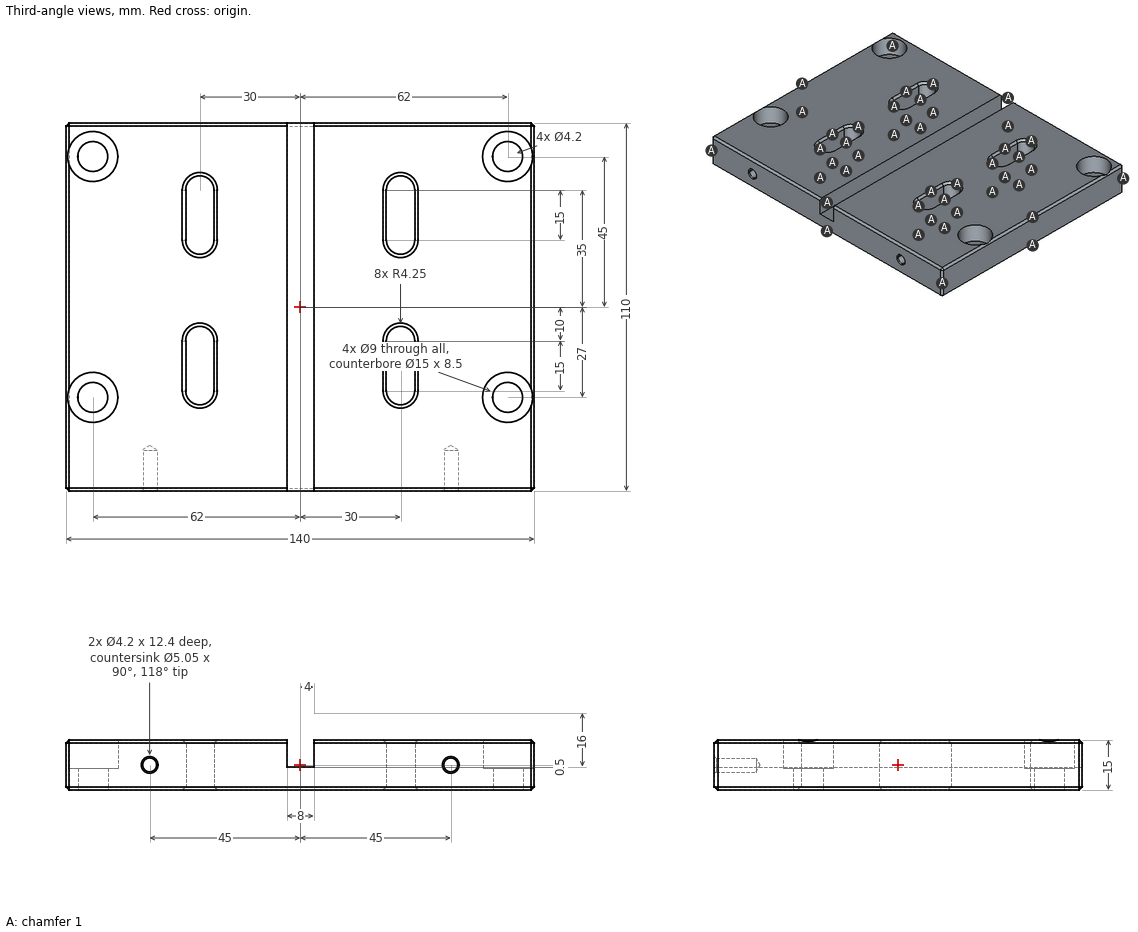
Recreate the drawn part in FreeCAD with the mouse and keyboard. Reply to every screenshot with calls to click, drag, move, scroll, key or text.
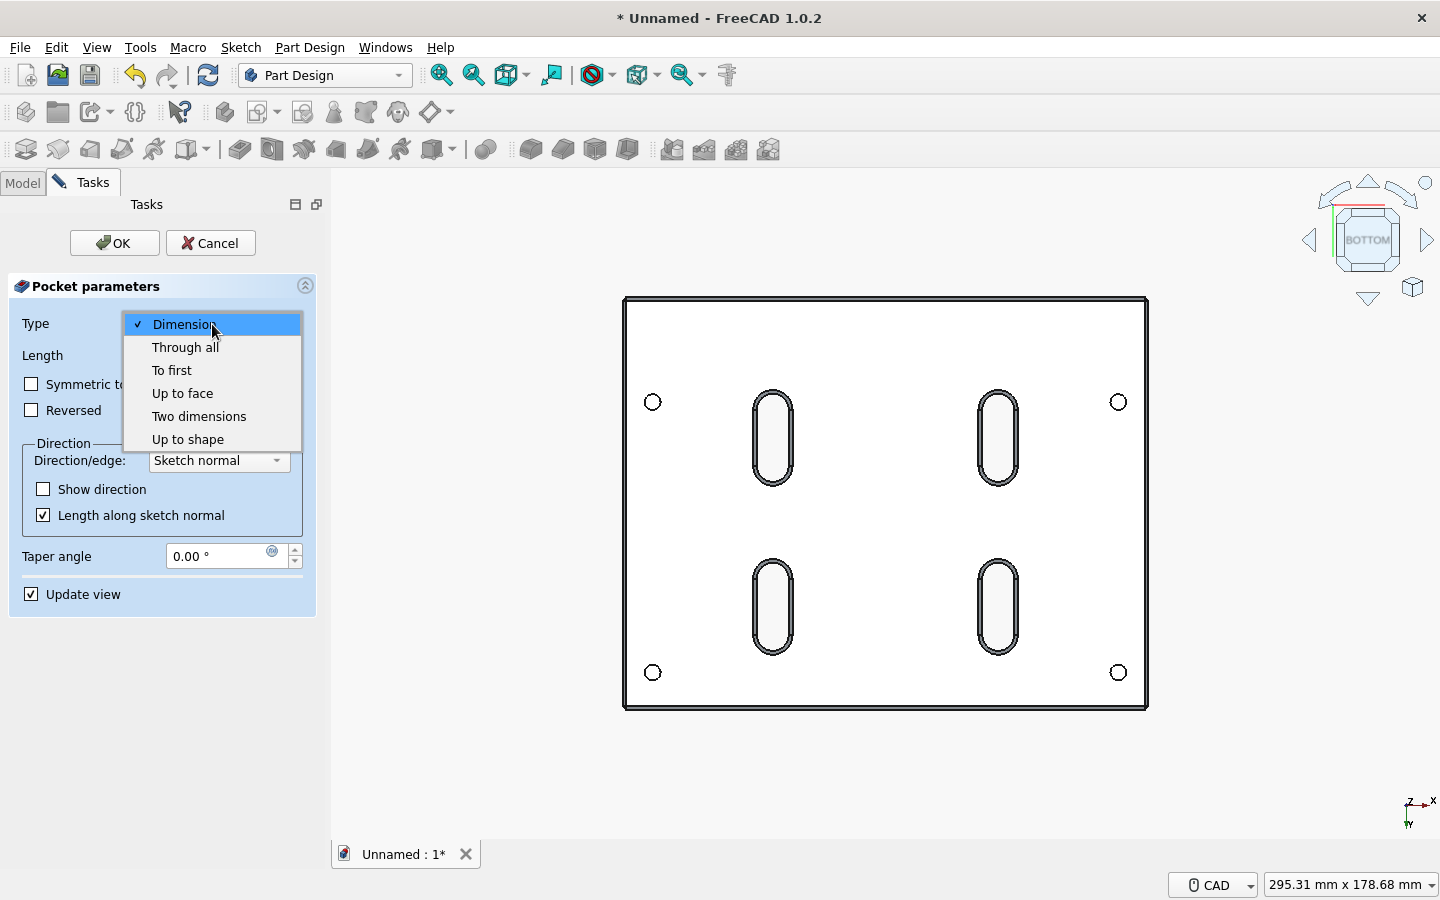
click(212, 348)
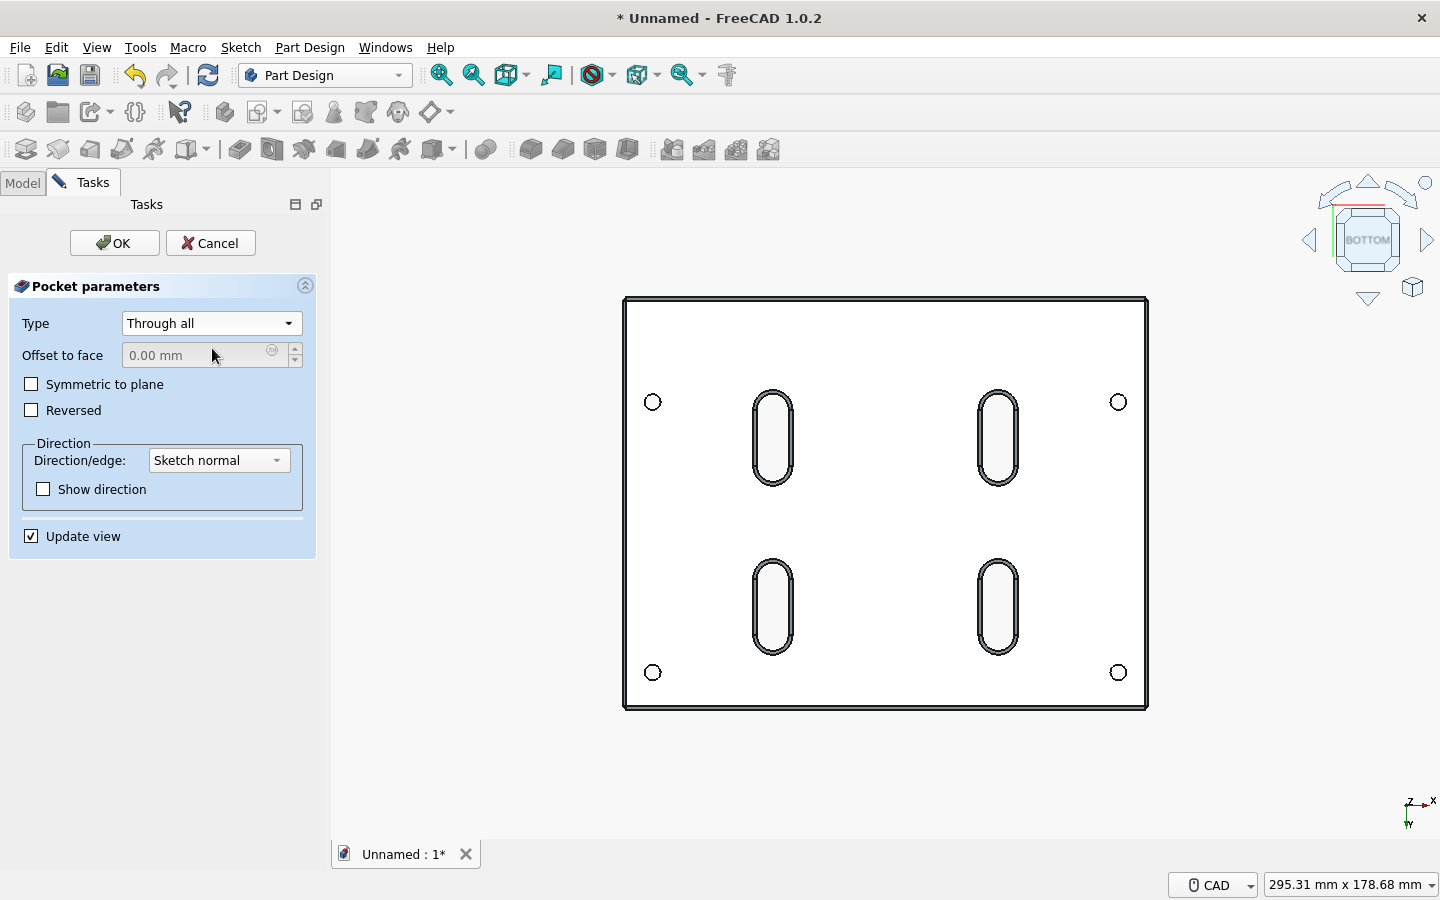
click(115, 243)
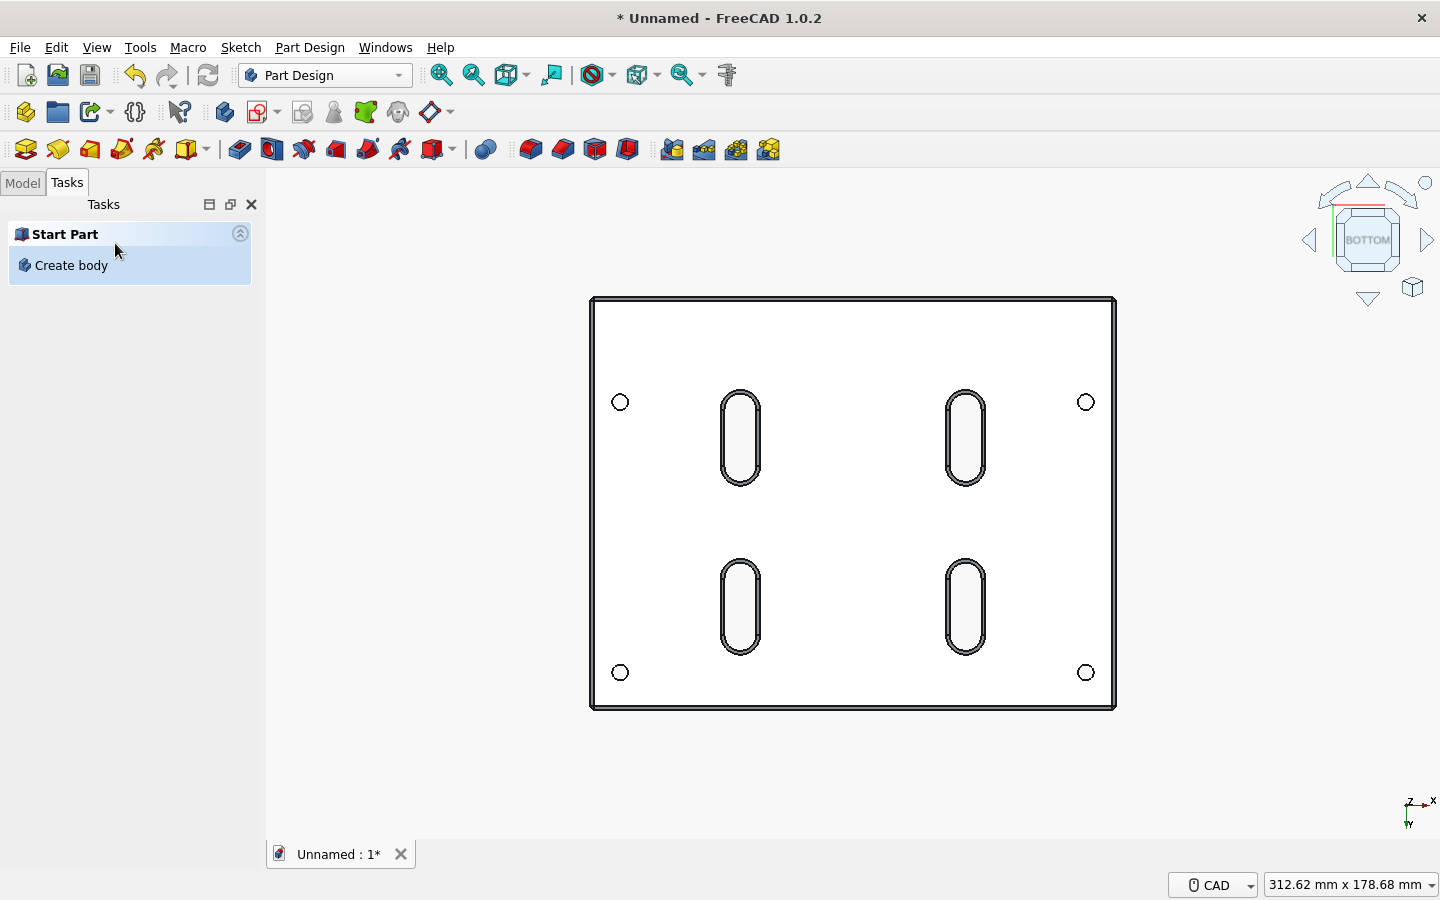
key(0)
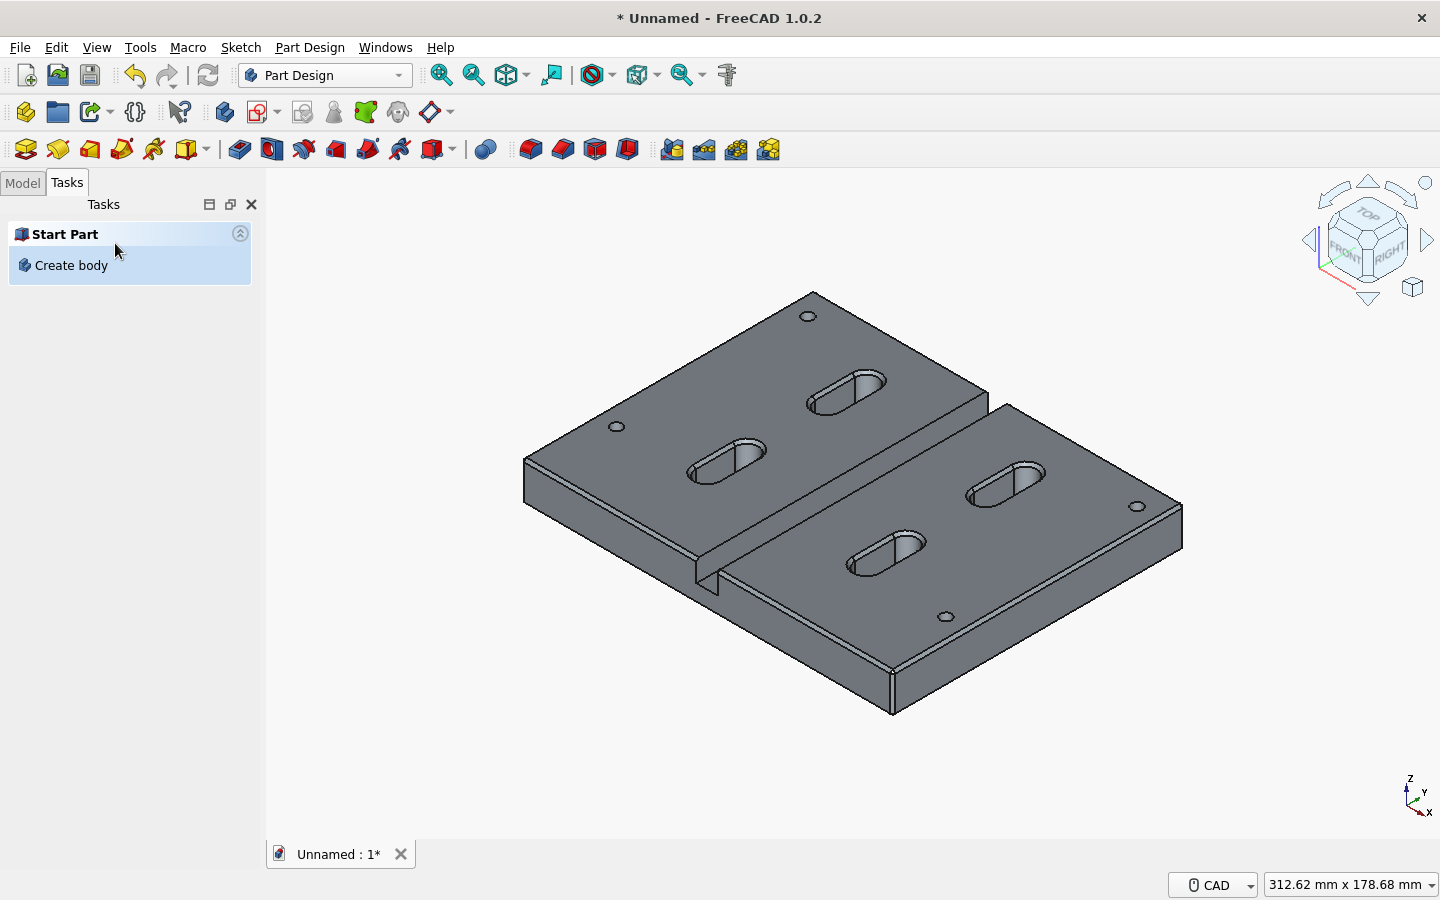
click(864, 677)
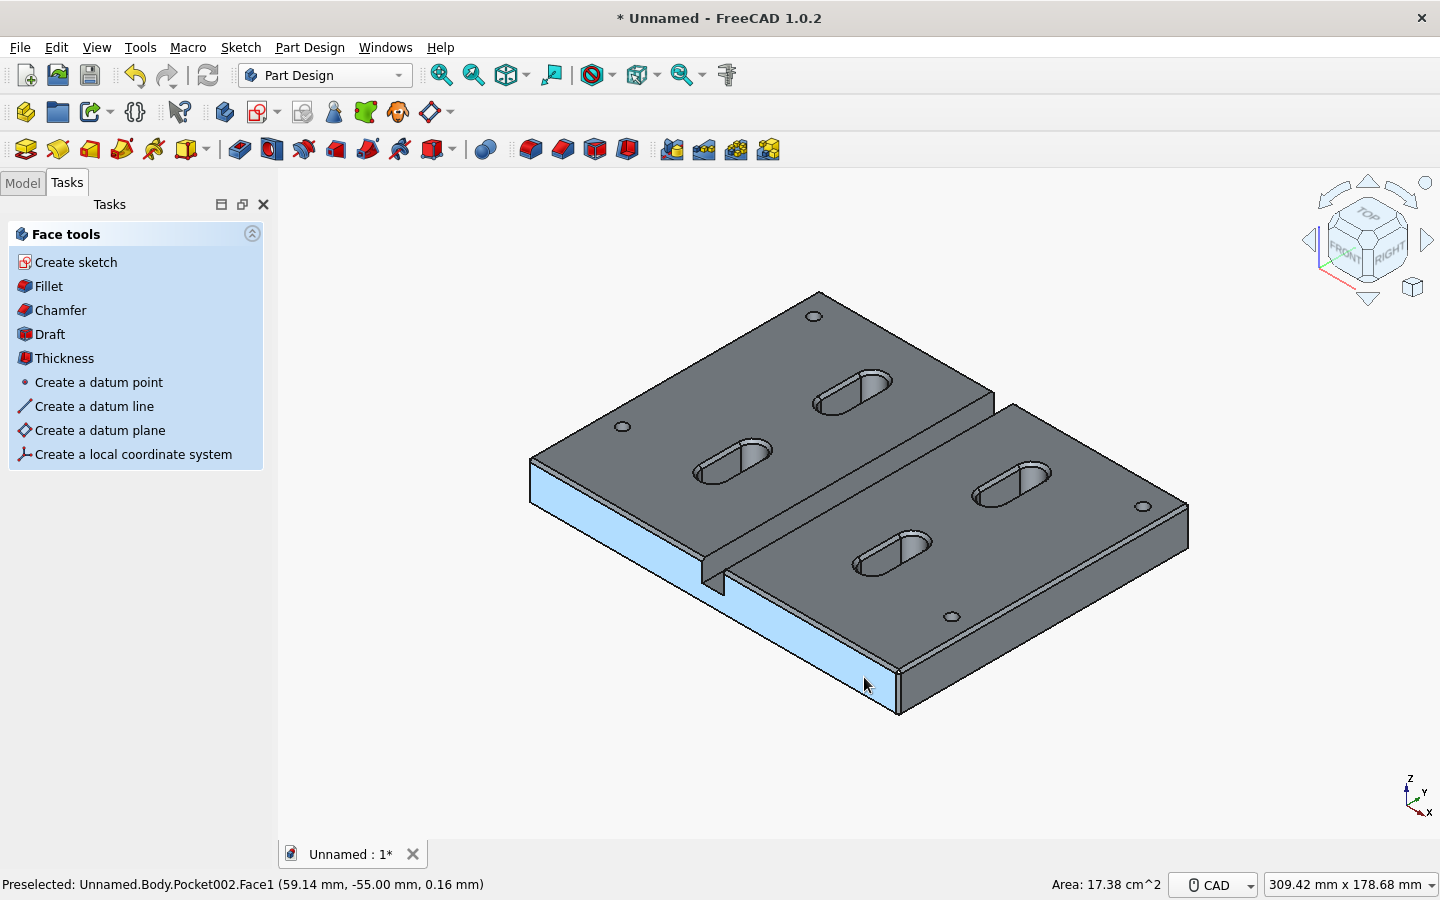
click(258, 112)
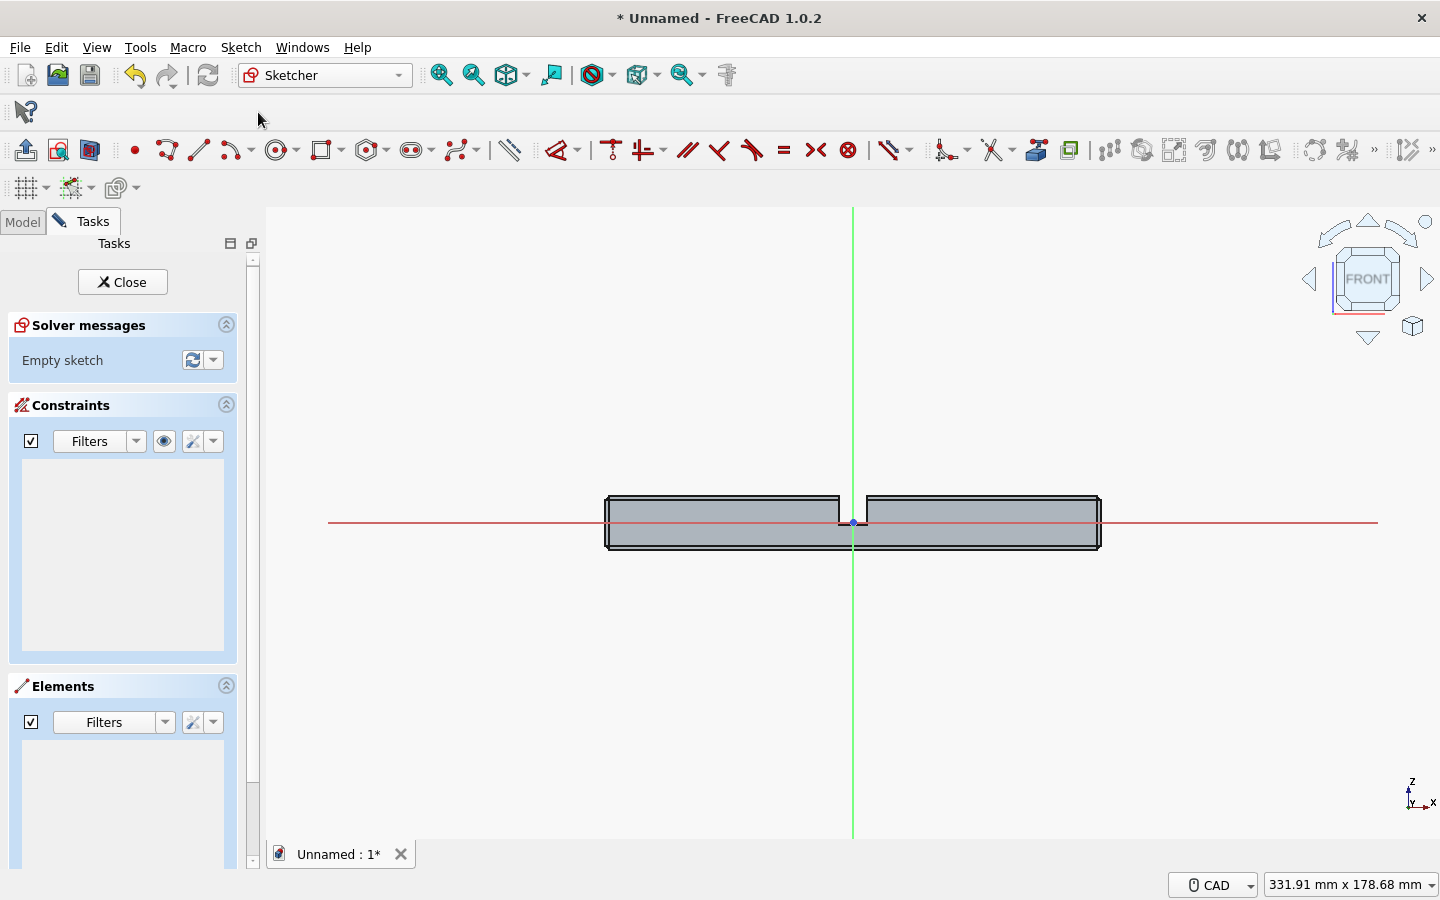
scroll(909, 523, up, 4)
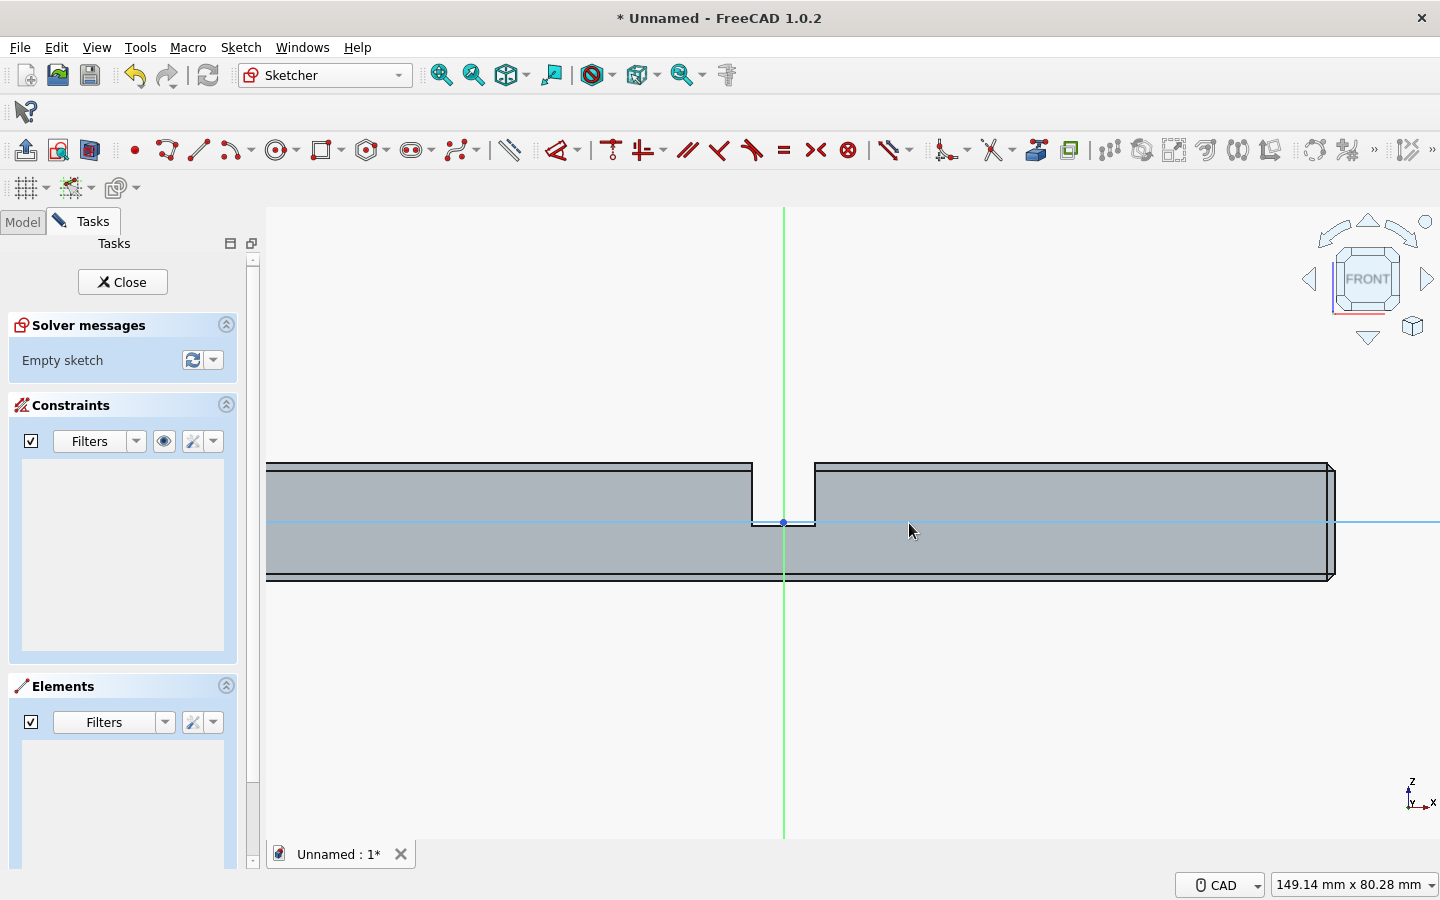
key(g)
key(c)